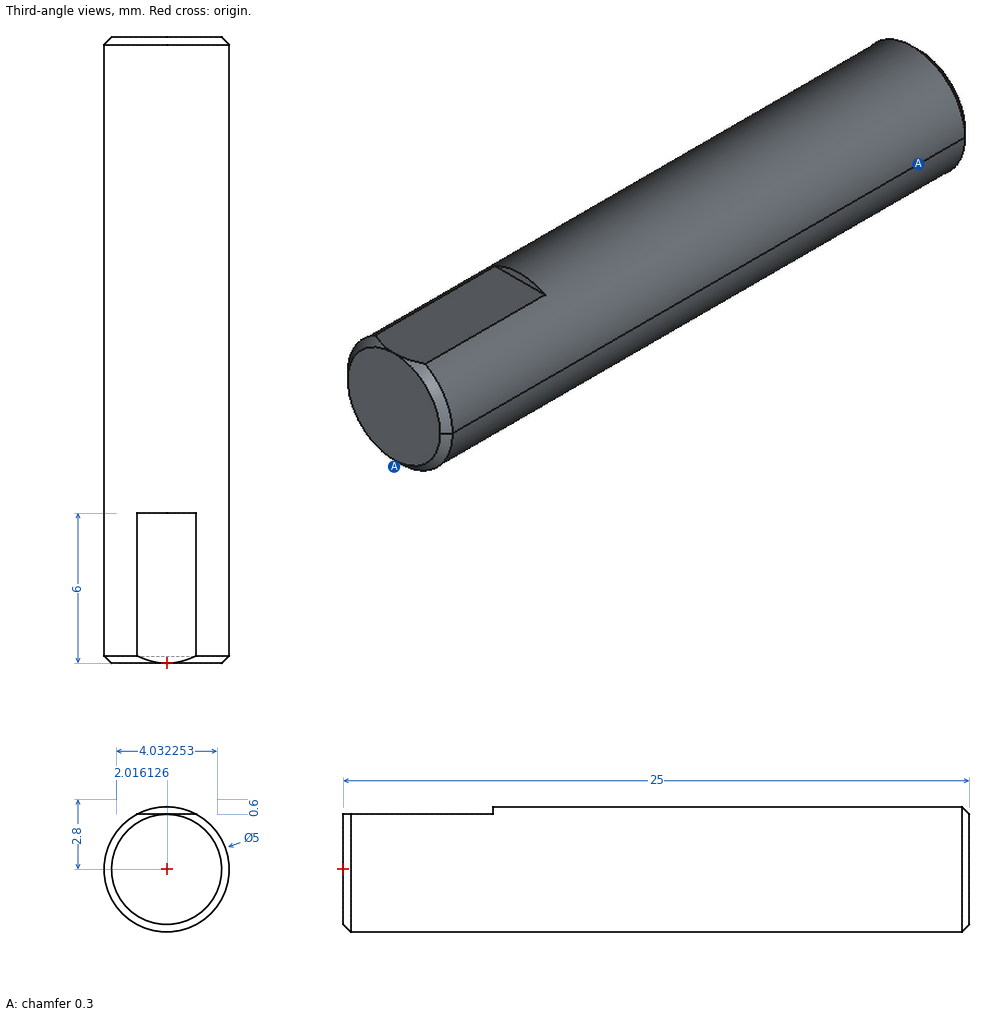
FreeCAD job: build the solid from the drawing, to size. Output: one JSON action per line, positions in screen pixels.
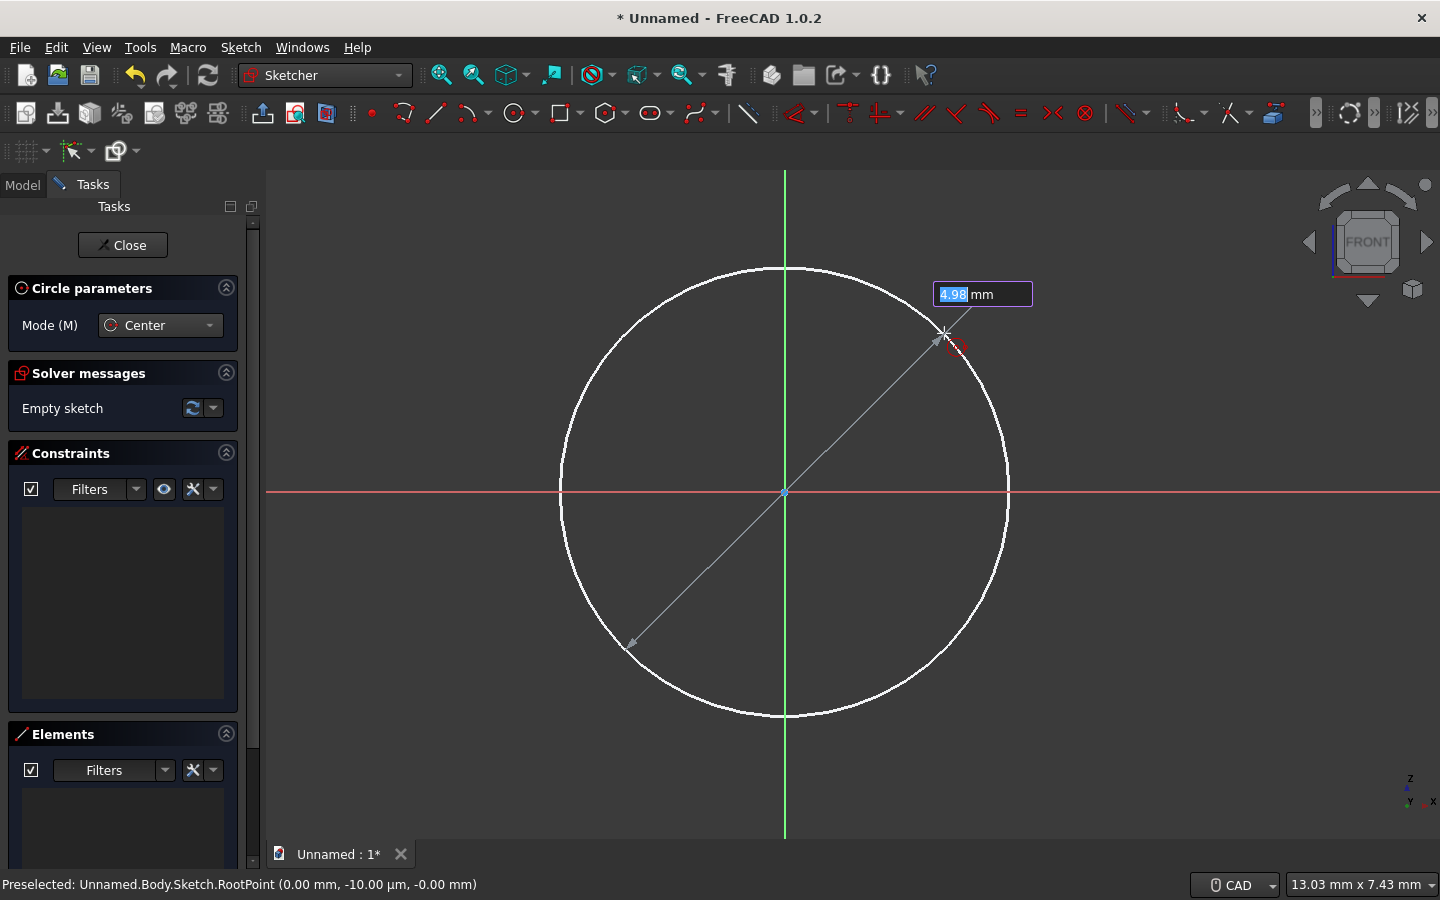
{"action": "type", "text": "5"}
{"action": "key", "text": "Return"}
{"action": "key", "text": "Escape"}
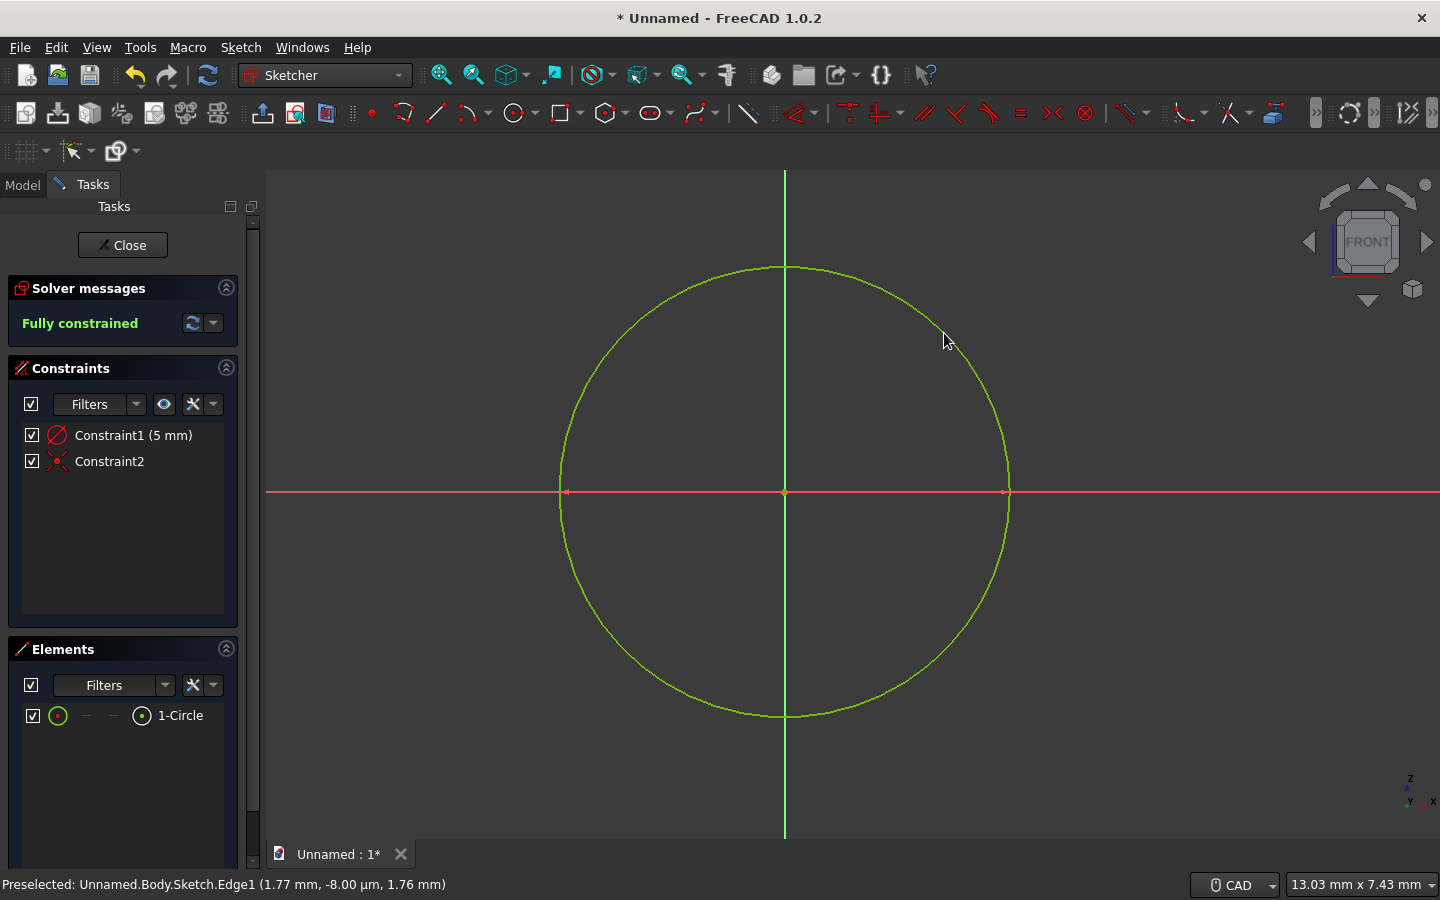
{"action": "left_click", "coordinate": [123, 245]}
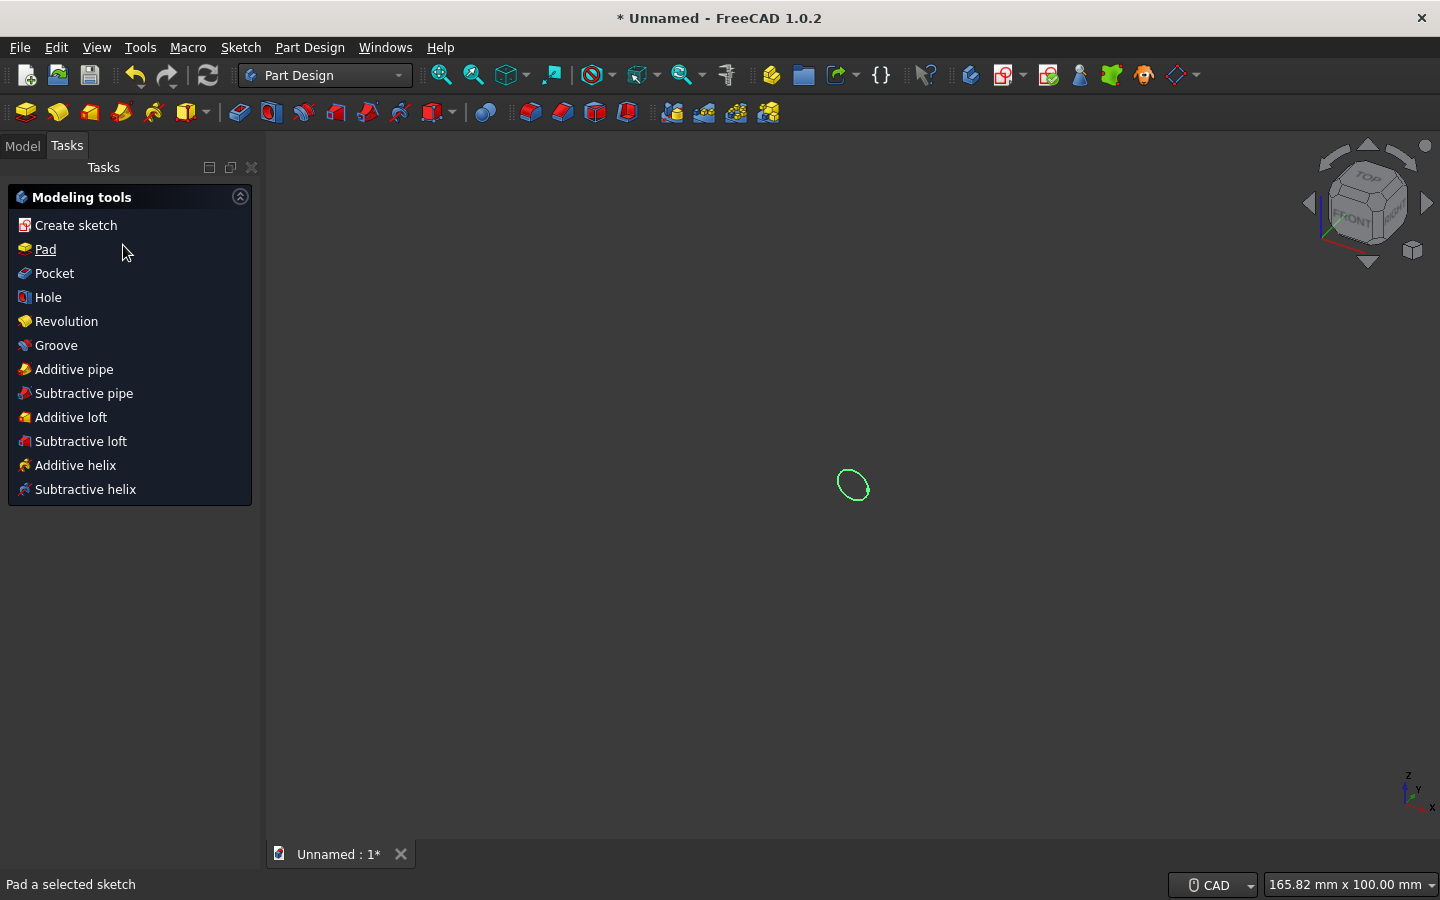
{"action": "left_click", "coordinate": [26, 112]}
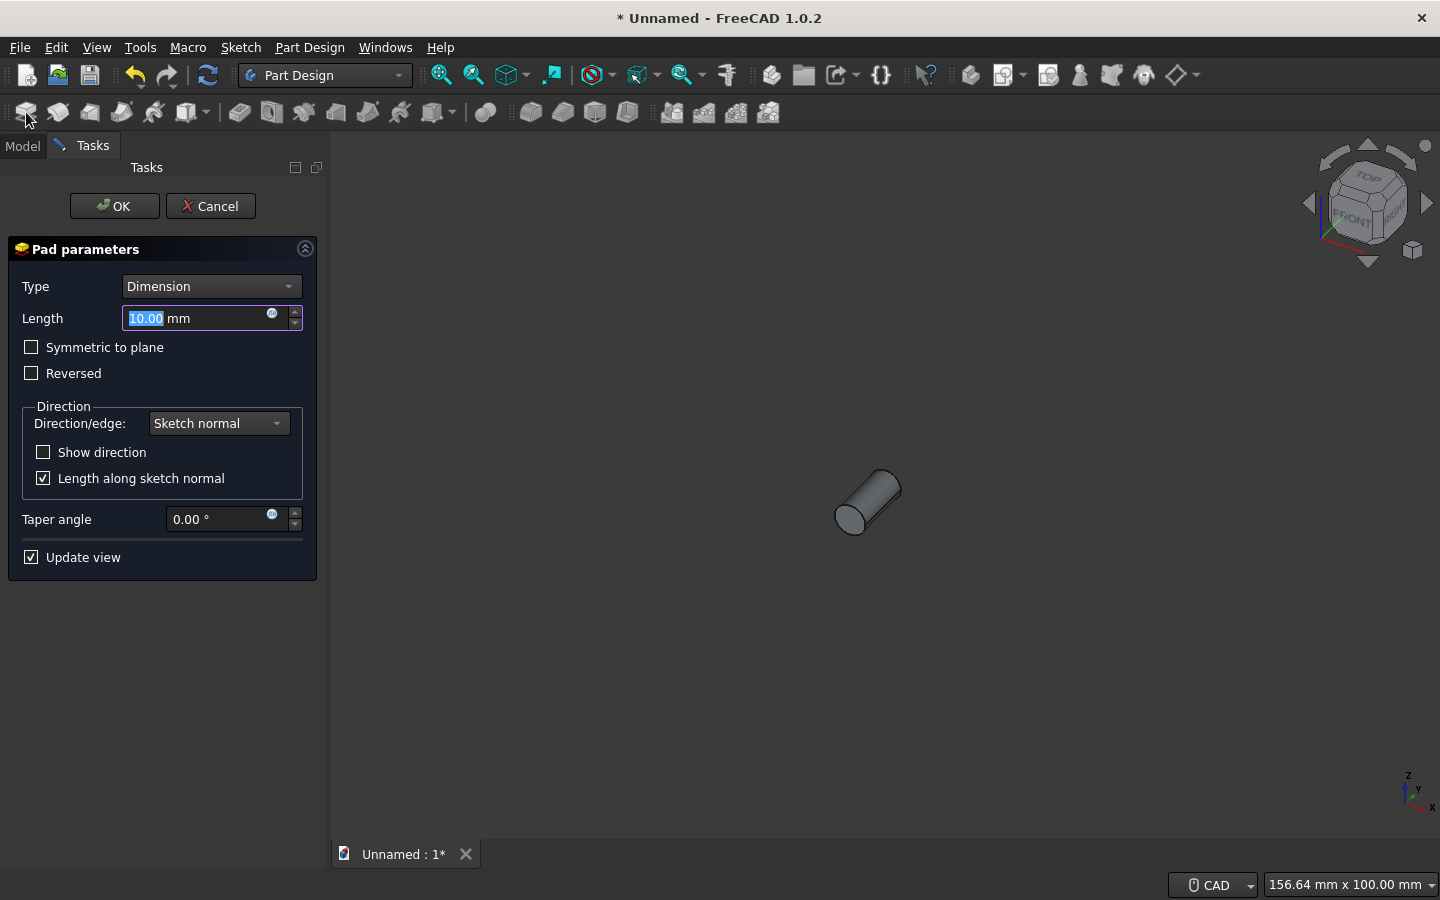
{"action": "type", "text": "25"}
{"action": "key", "text": "Tab"}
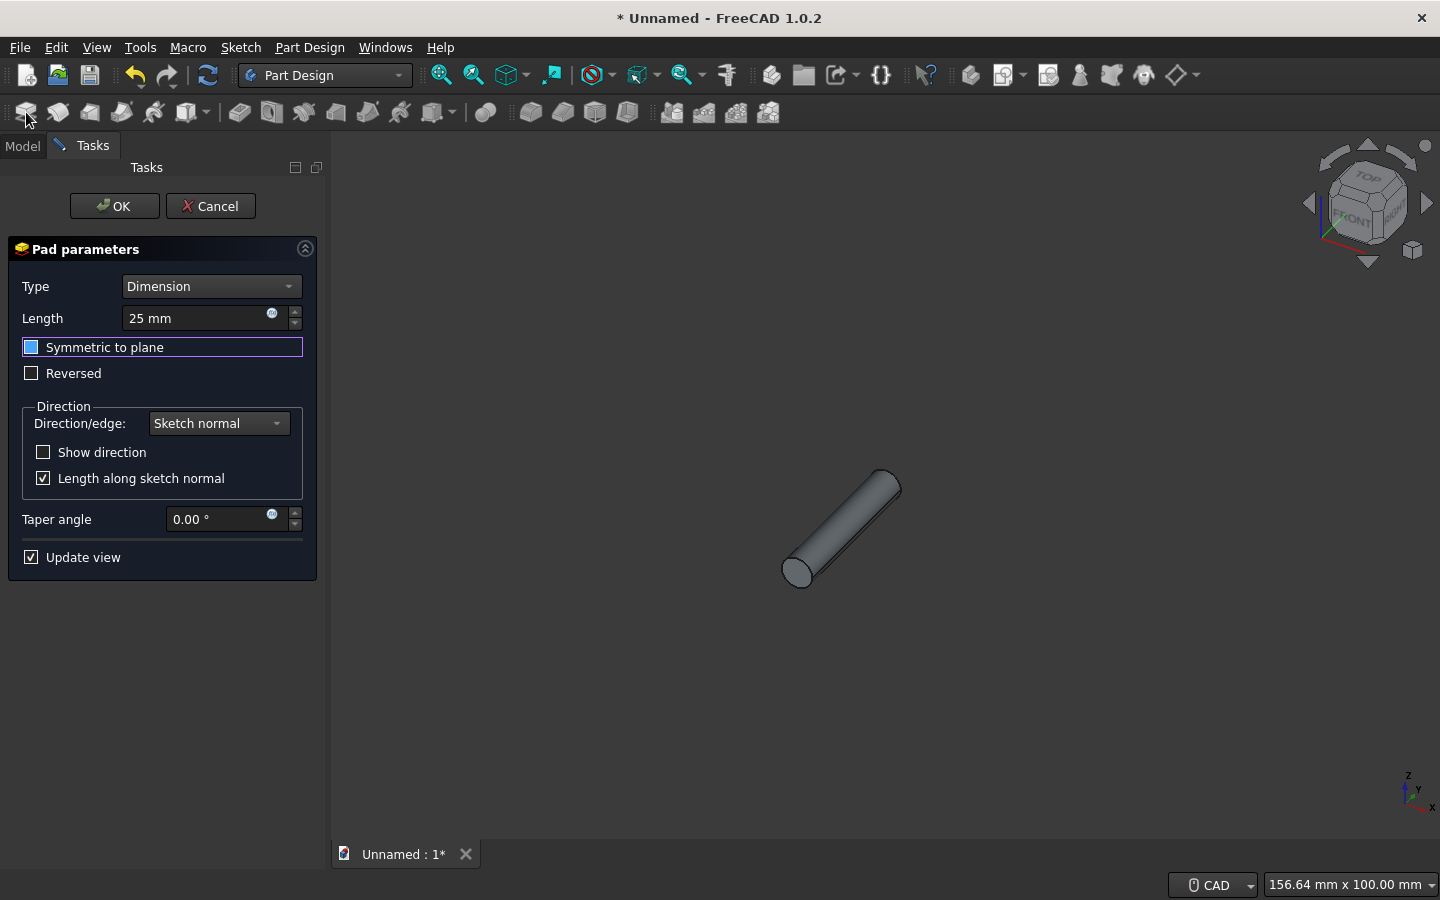
{"action": "left_click", "coordinate": [30, 373]}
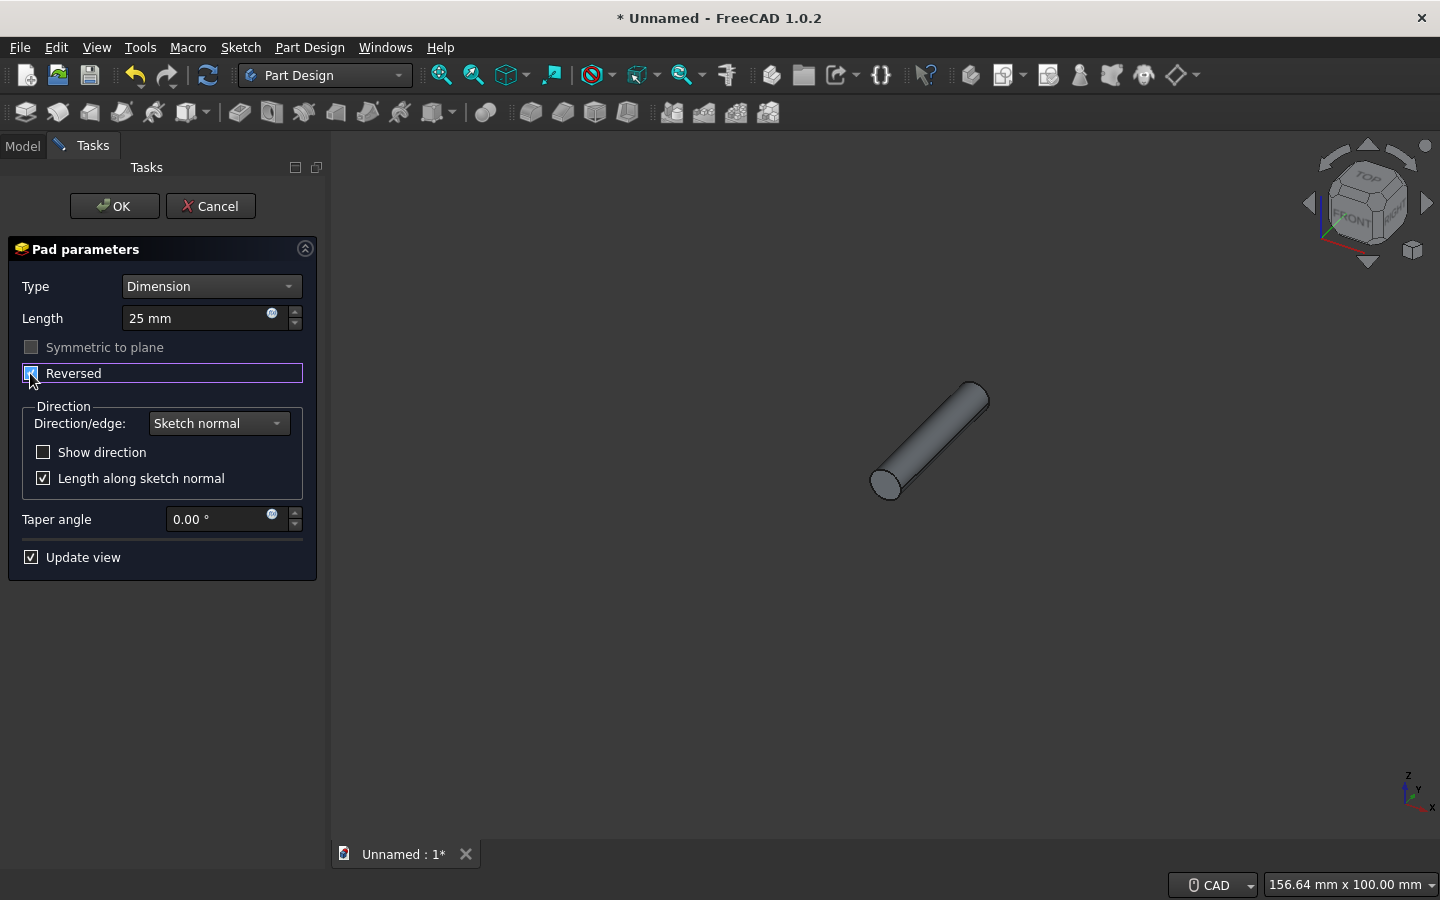
{"action": "left_click", "coordinate": [115, 206]}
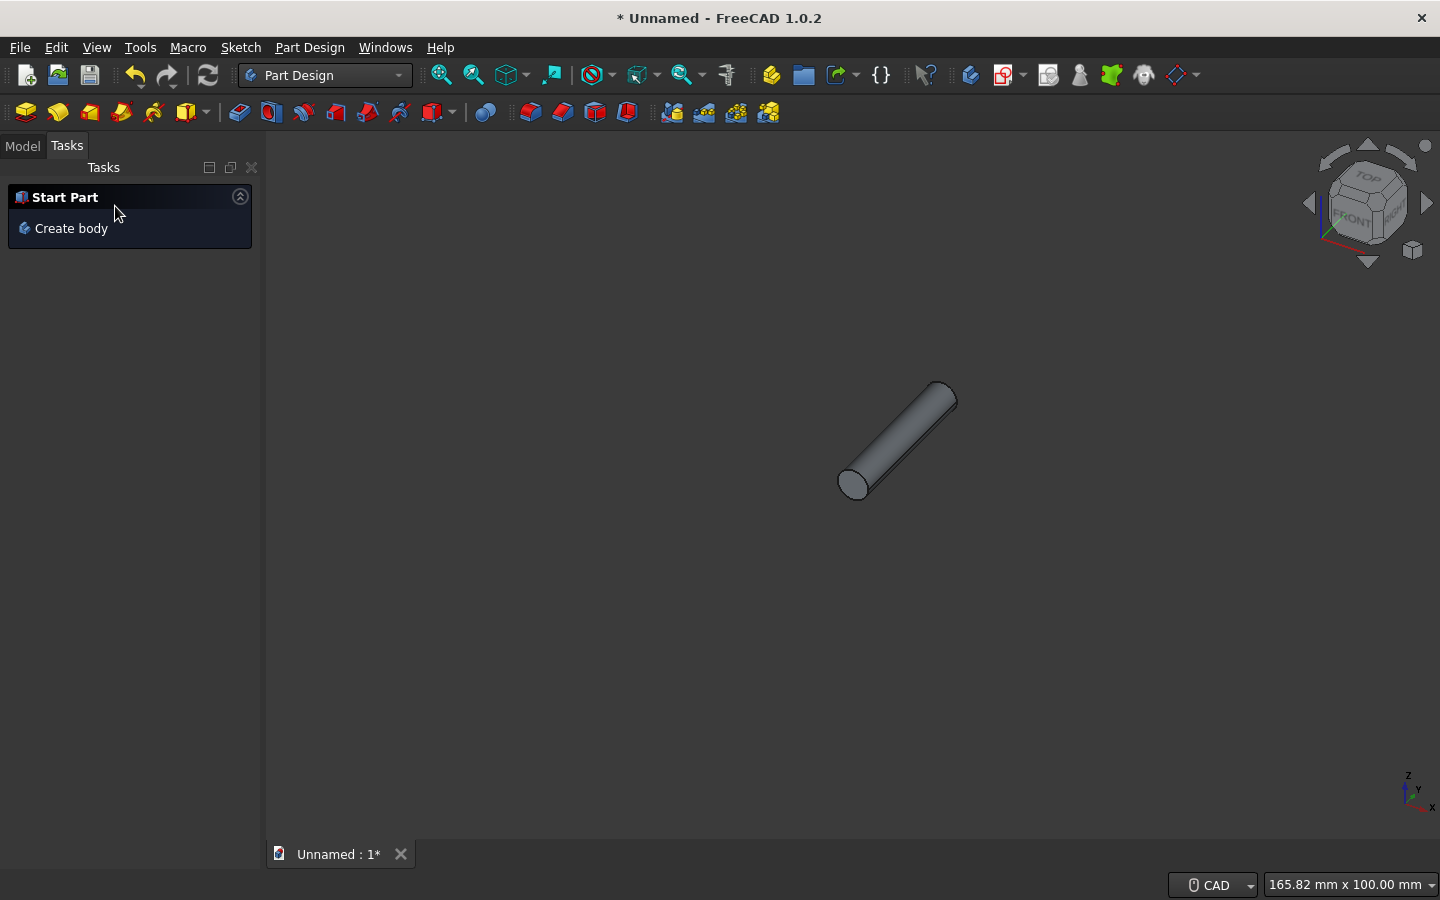
{"action": "left_click", "coordinate": [442, 76]}